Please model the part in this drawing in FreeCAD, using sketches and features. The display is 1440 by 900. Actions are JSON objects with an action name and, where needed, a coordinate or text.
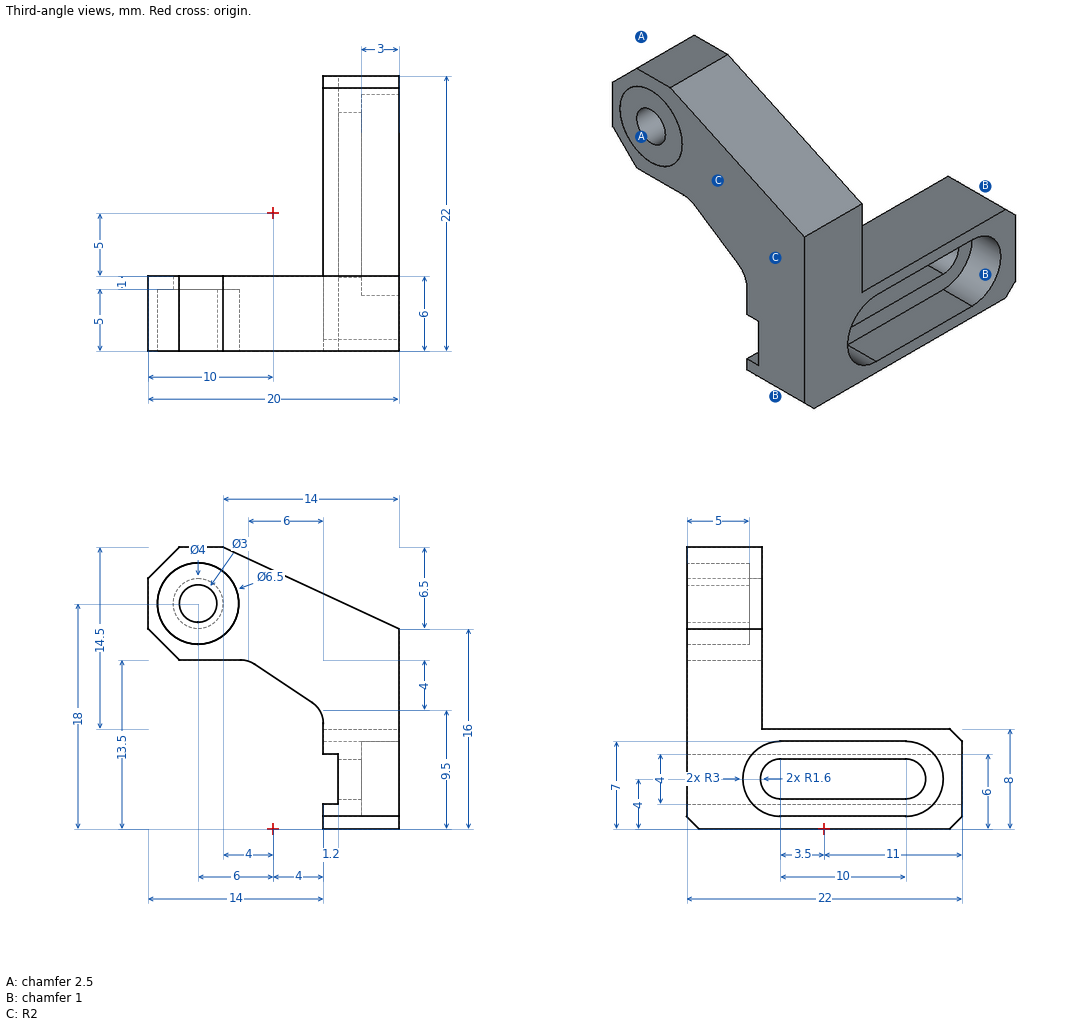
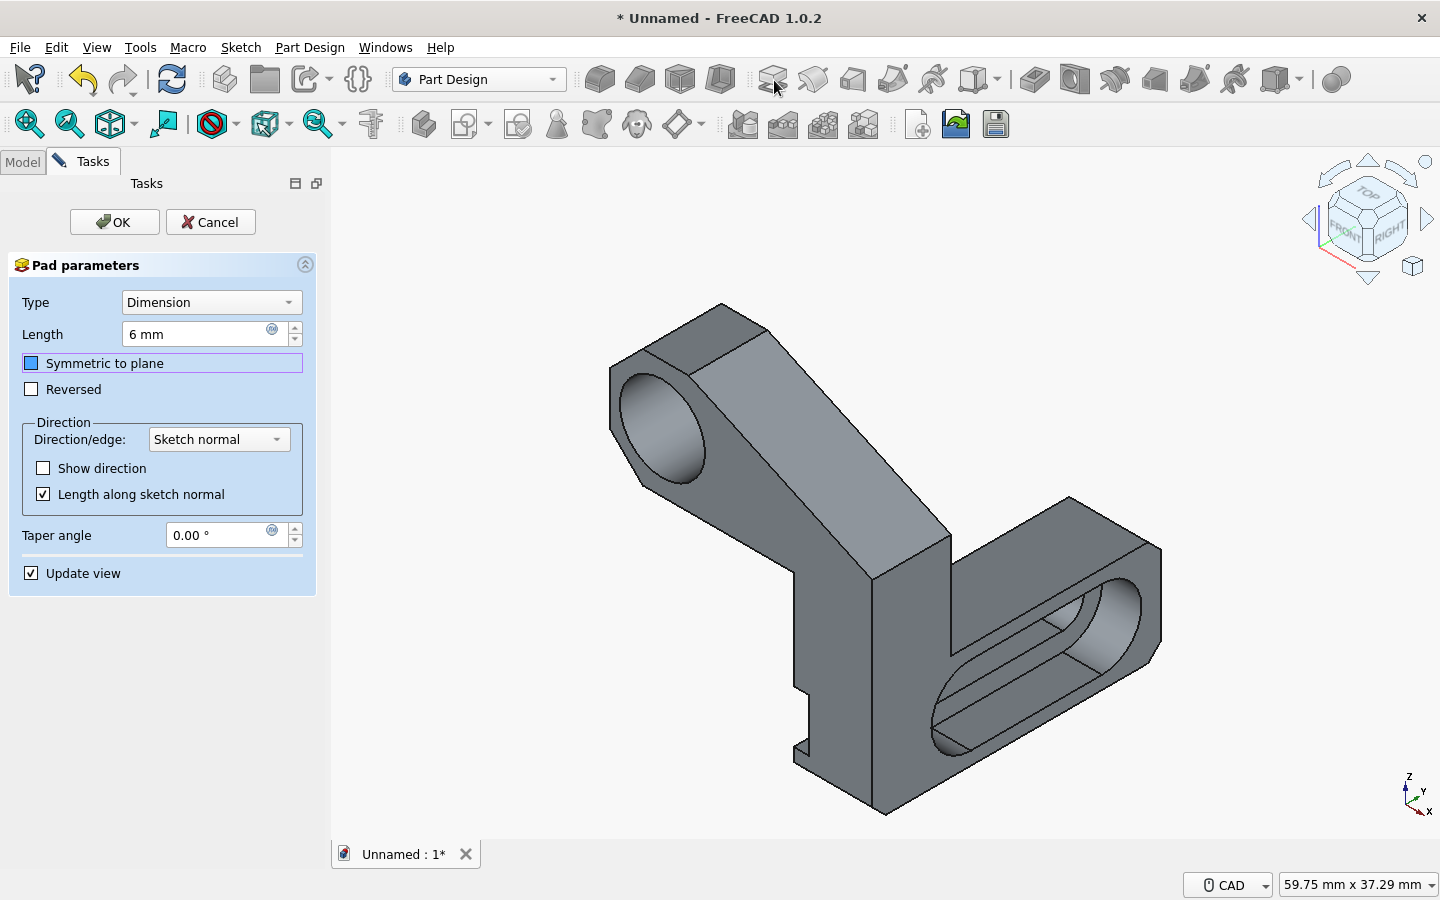
{"action": "left_click", "coordinate": [30, 389]}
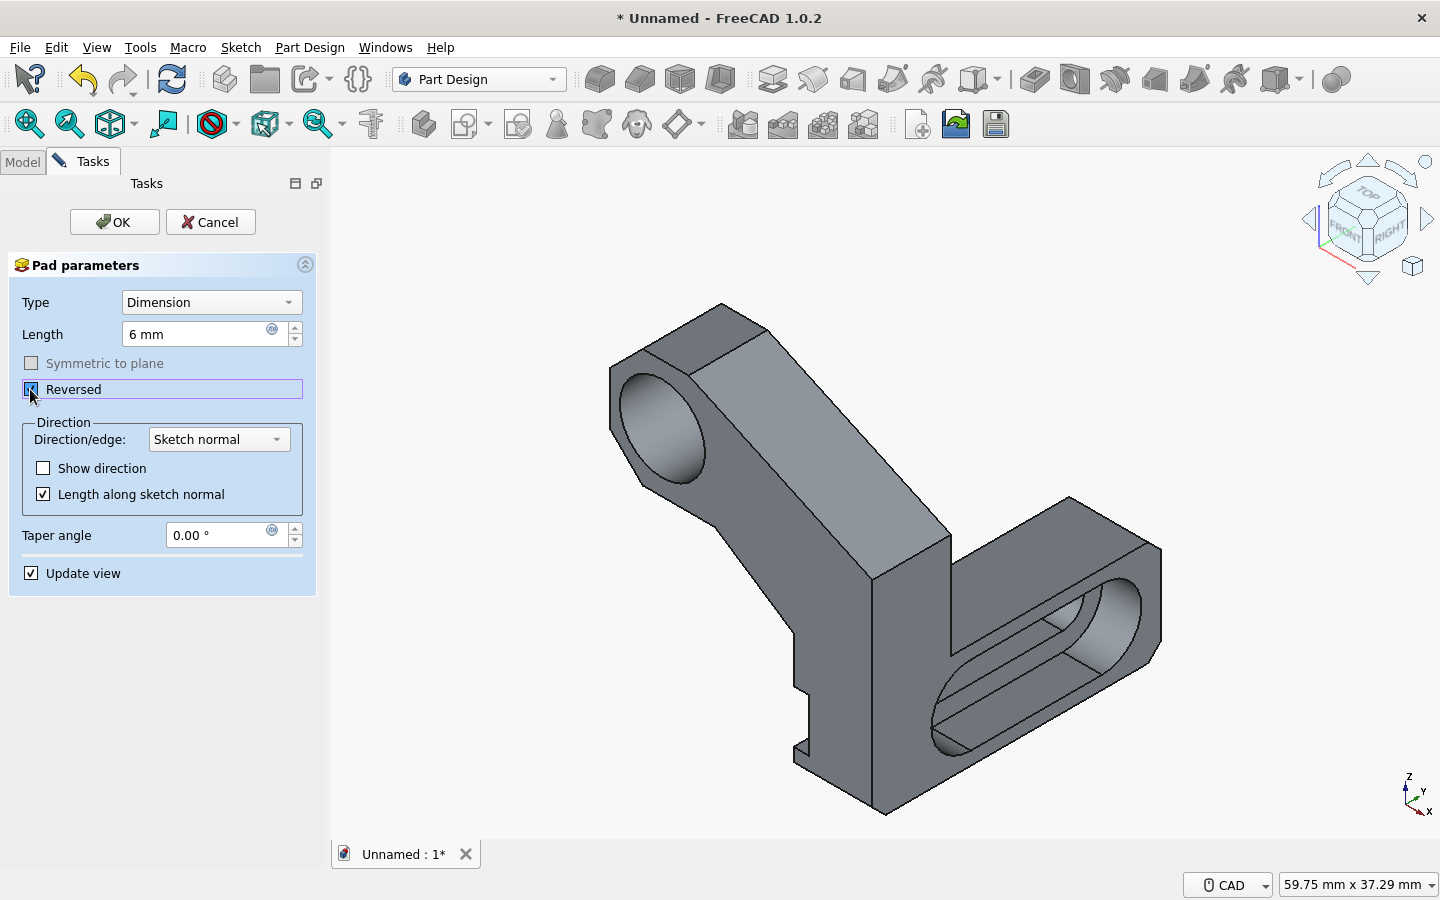
{"action": "left_click", "coordinate": [115, 222]}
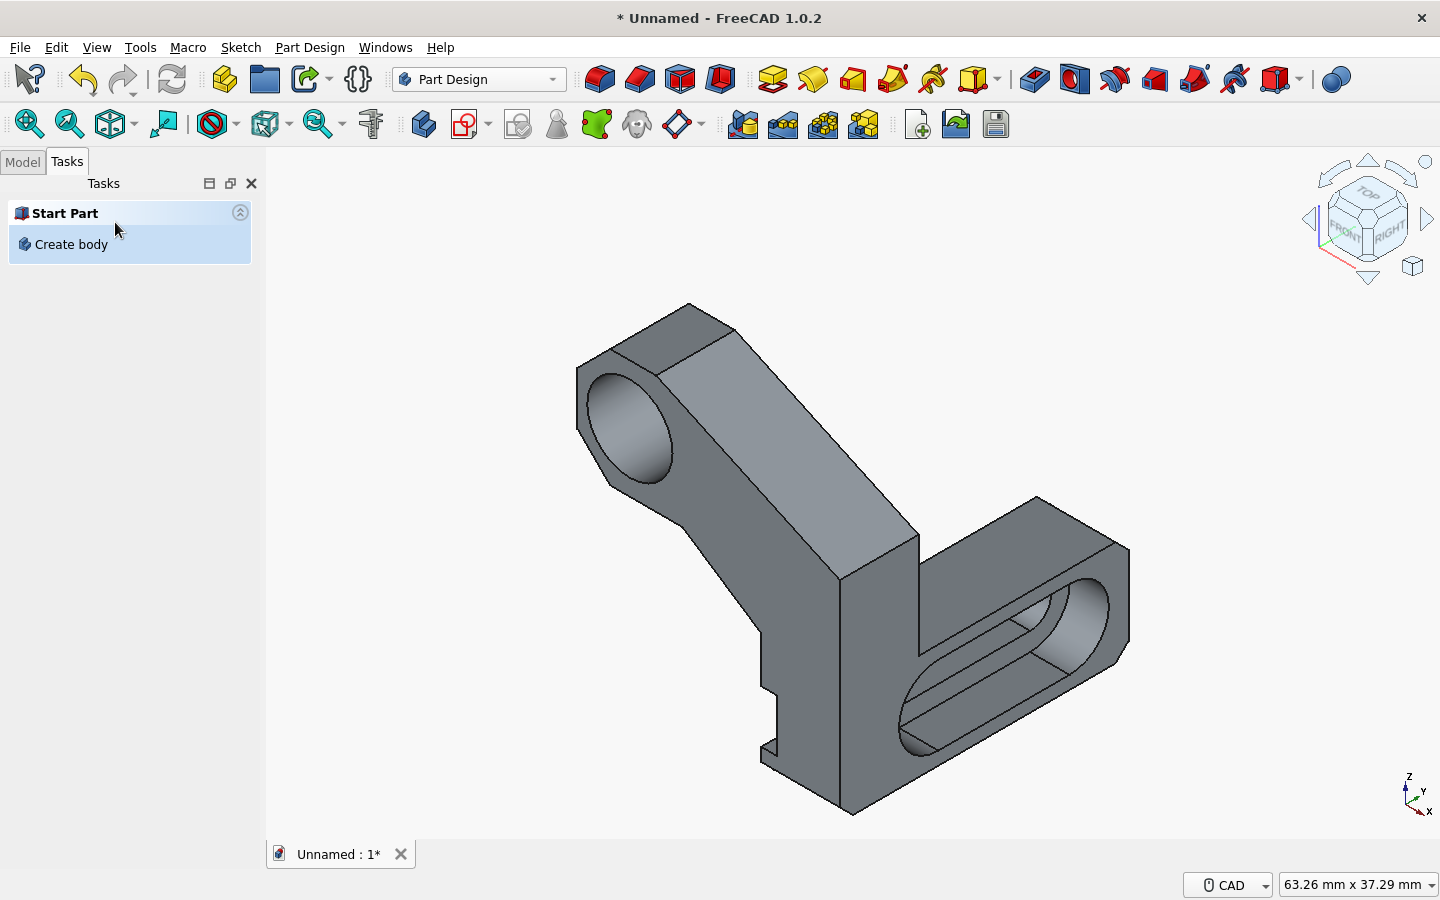
{"action": "key", "text": "2"}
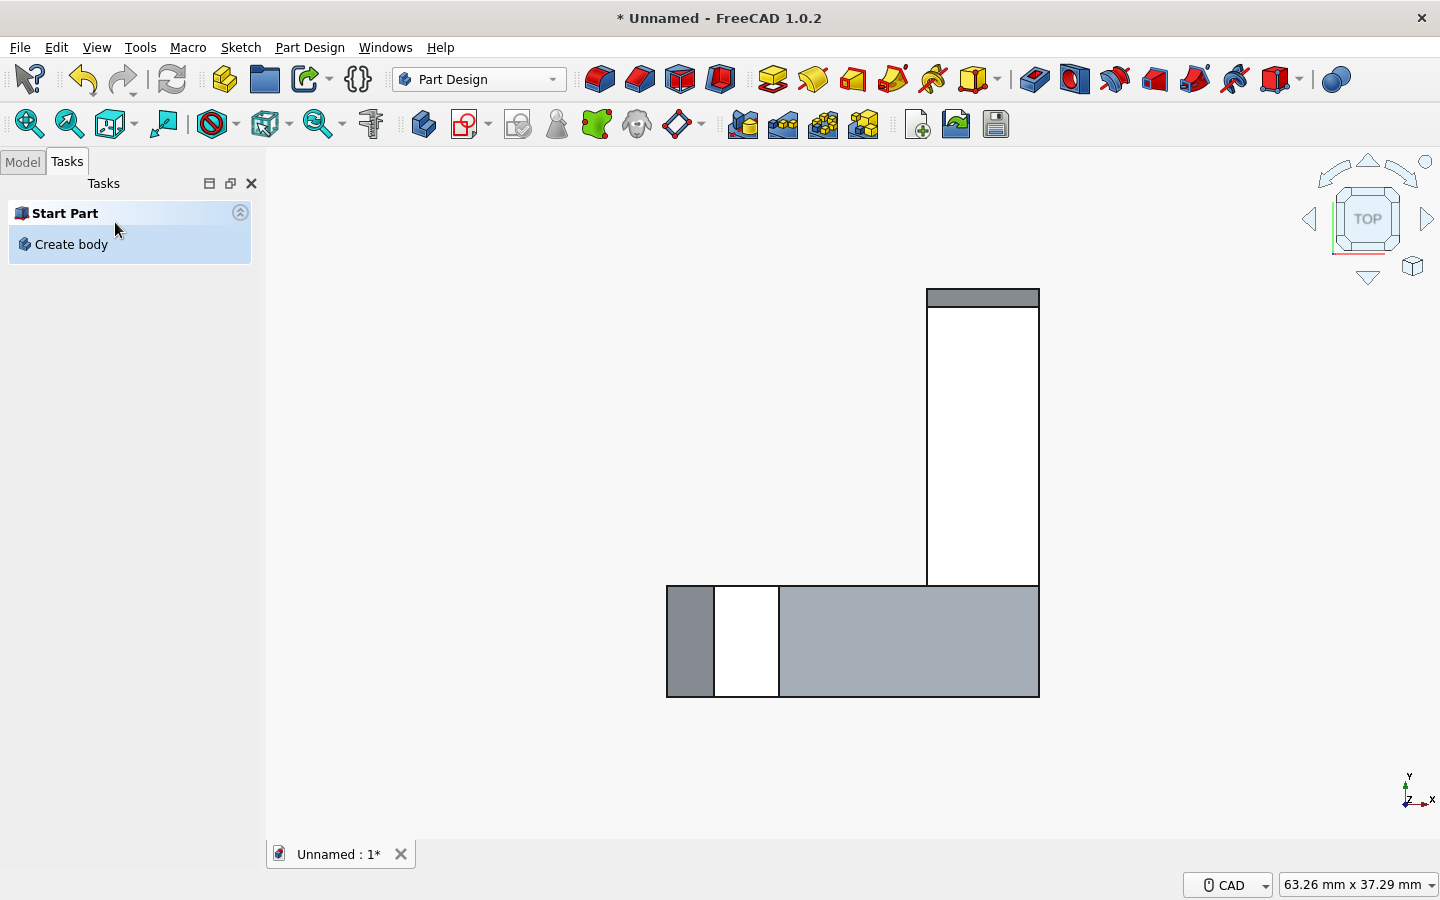
{"action": "key", "text": "0"}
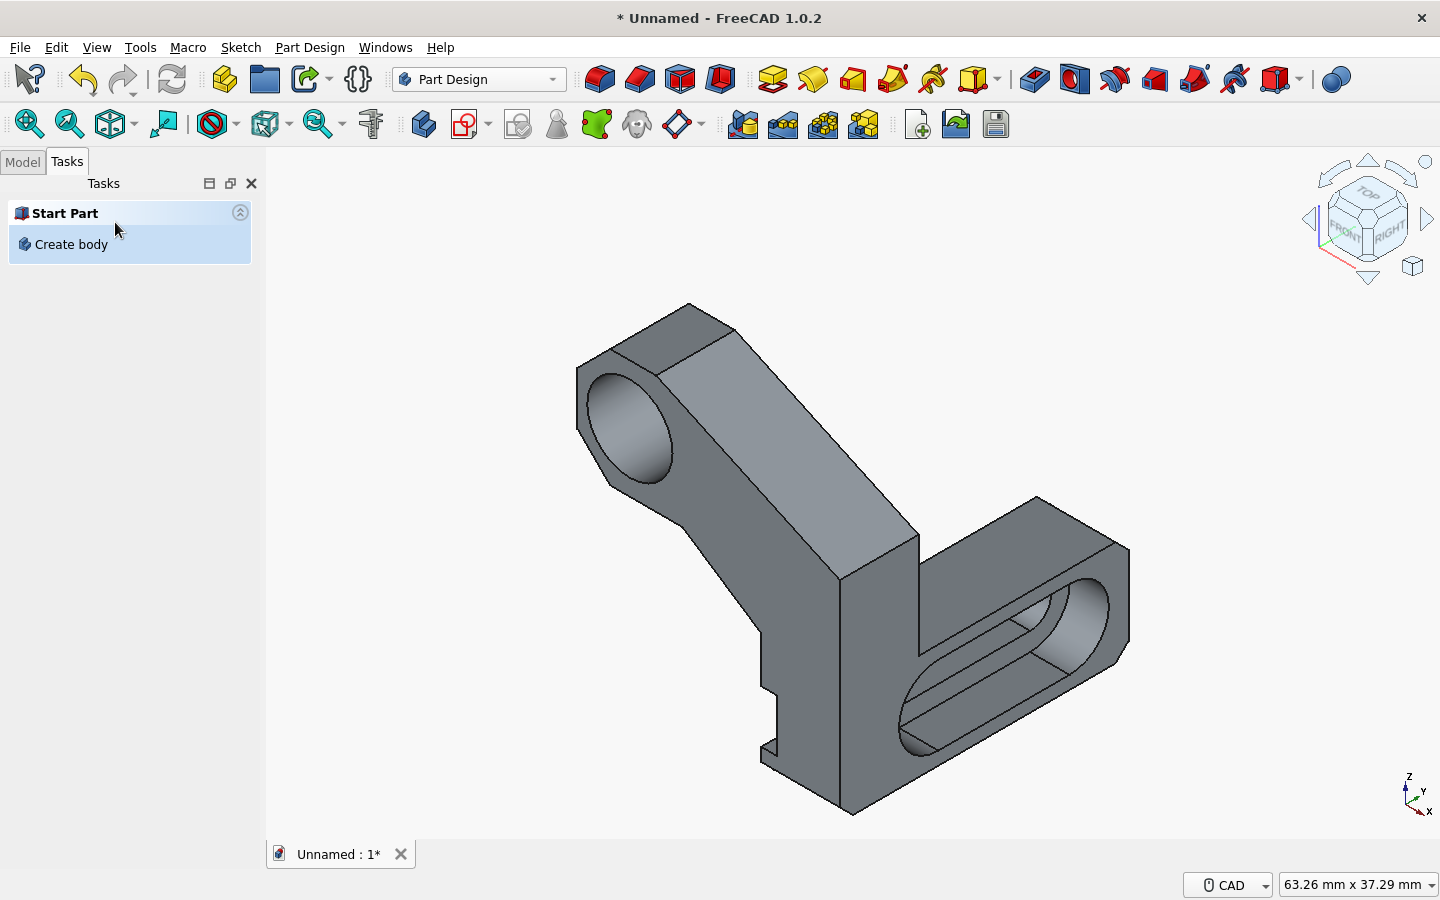
{"action": "key", "text": "1"}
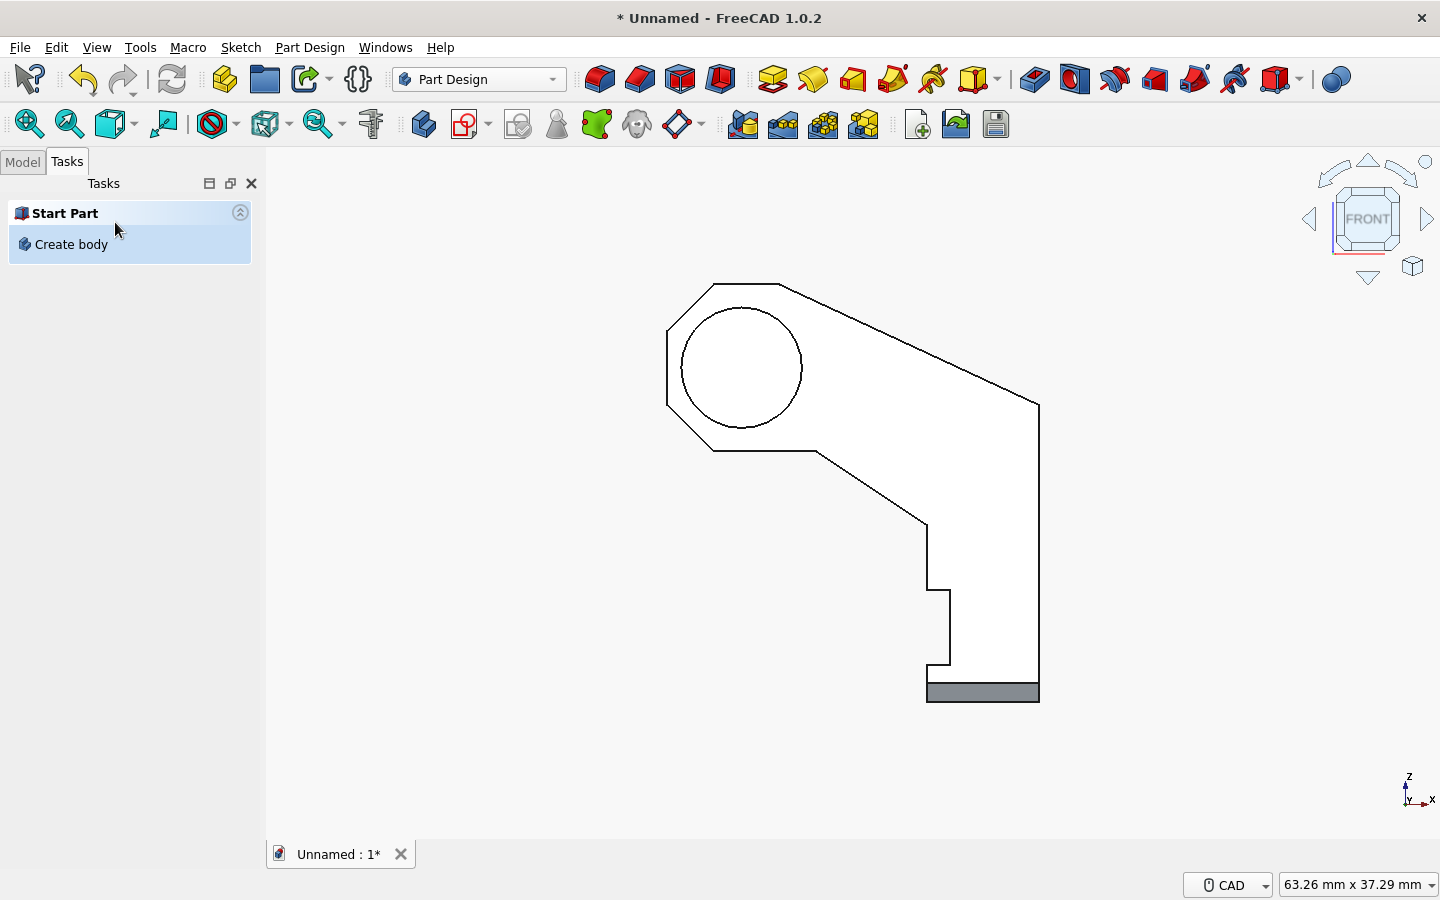
{"action": "key", "text": "3"}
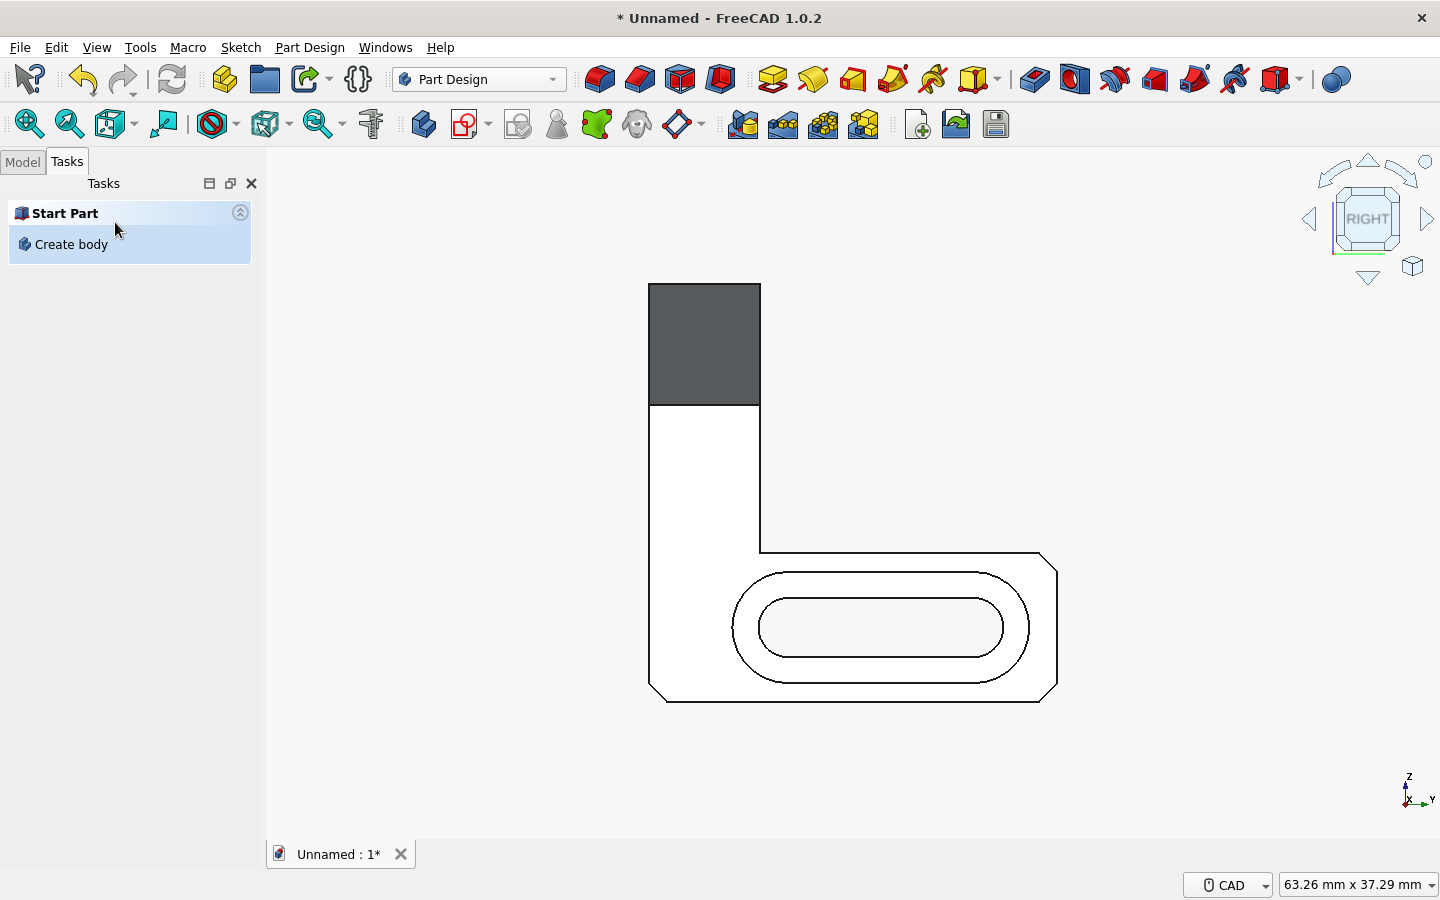
{"action": "key", "text": "5"}